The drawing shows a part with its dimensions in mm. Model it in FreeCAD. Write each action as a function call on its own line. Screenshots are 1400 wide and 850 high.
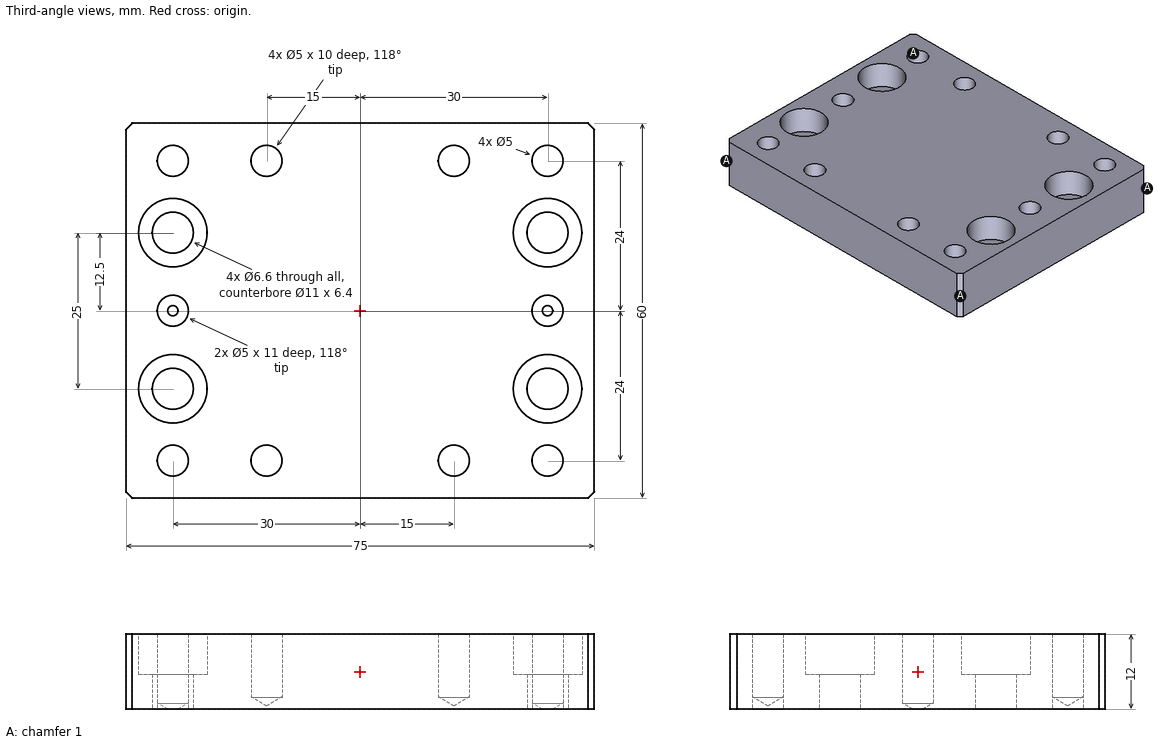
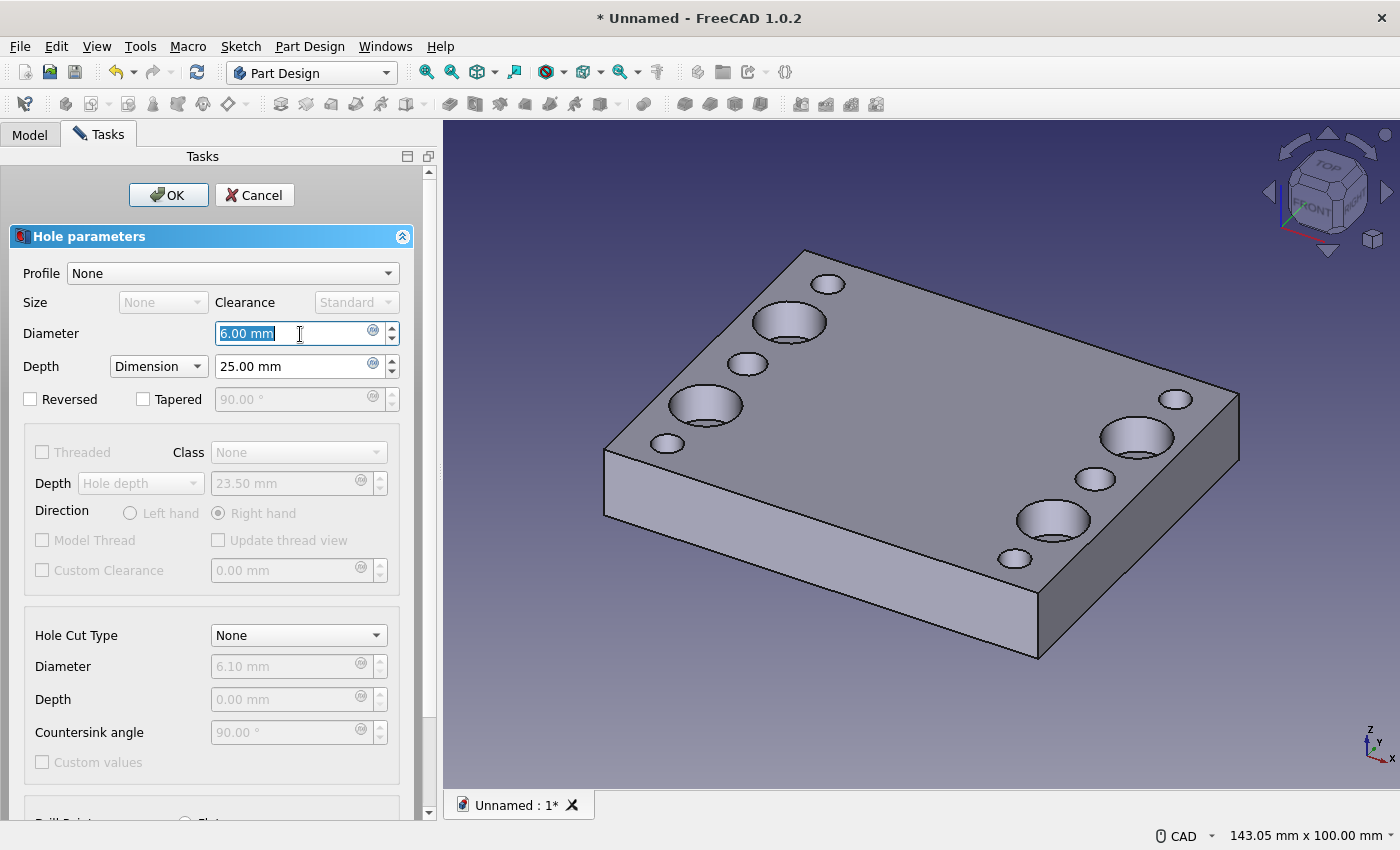
text(5)
key(Tab)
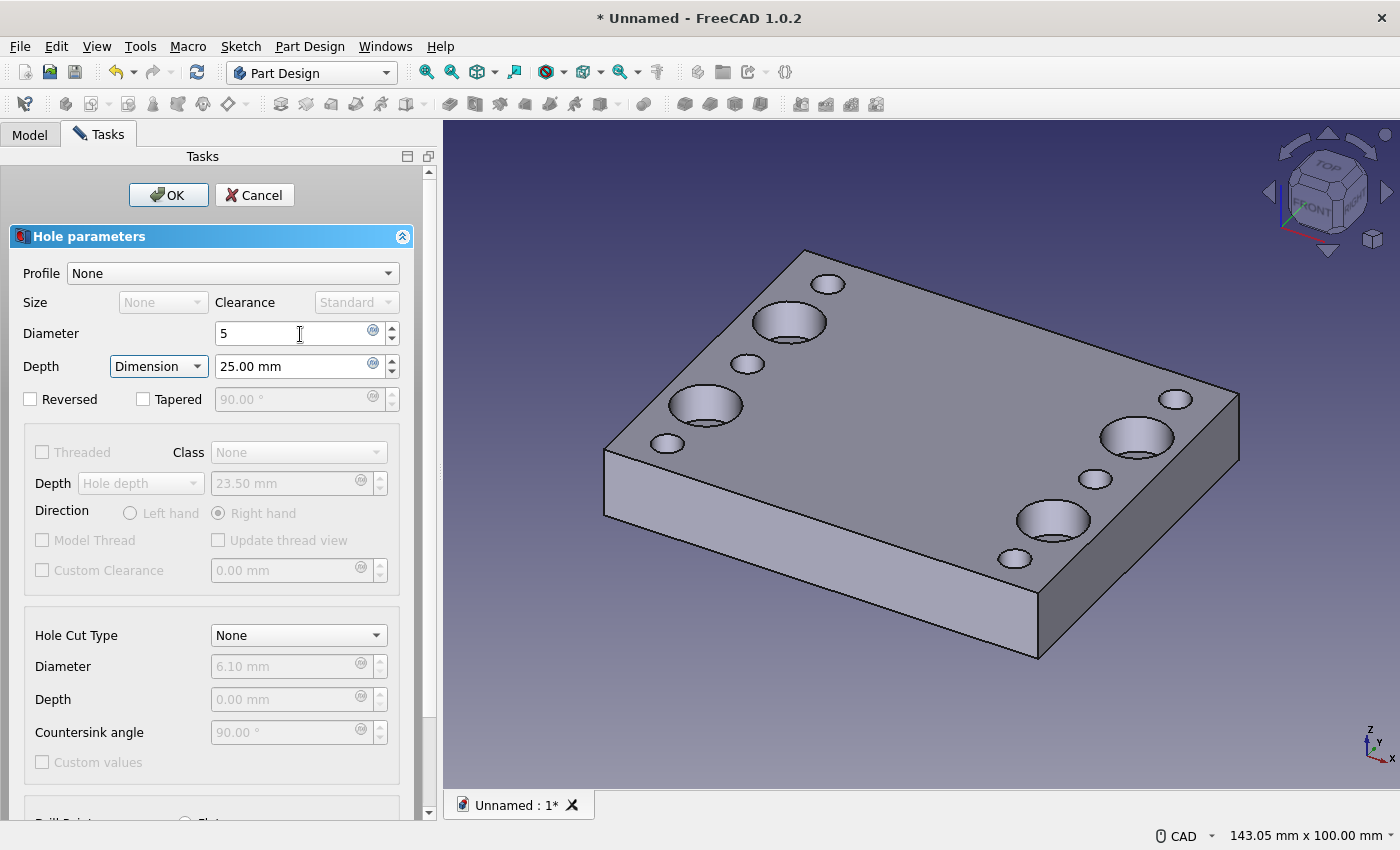
triple_click(300, 366)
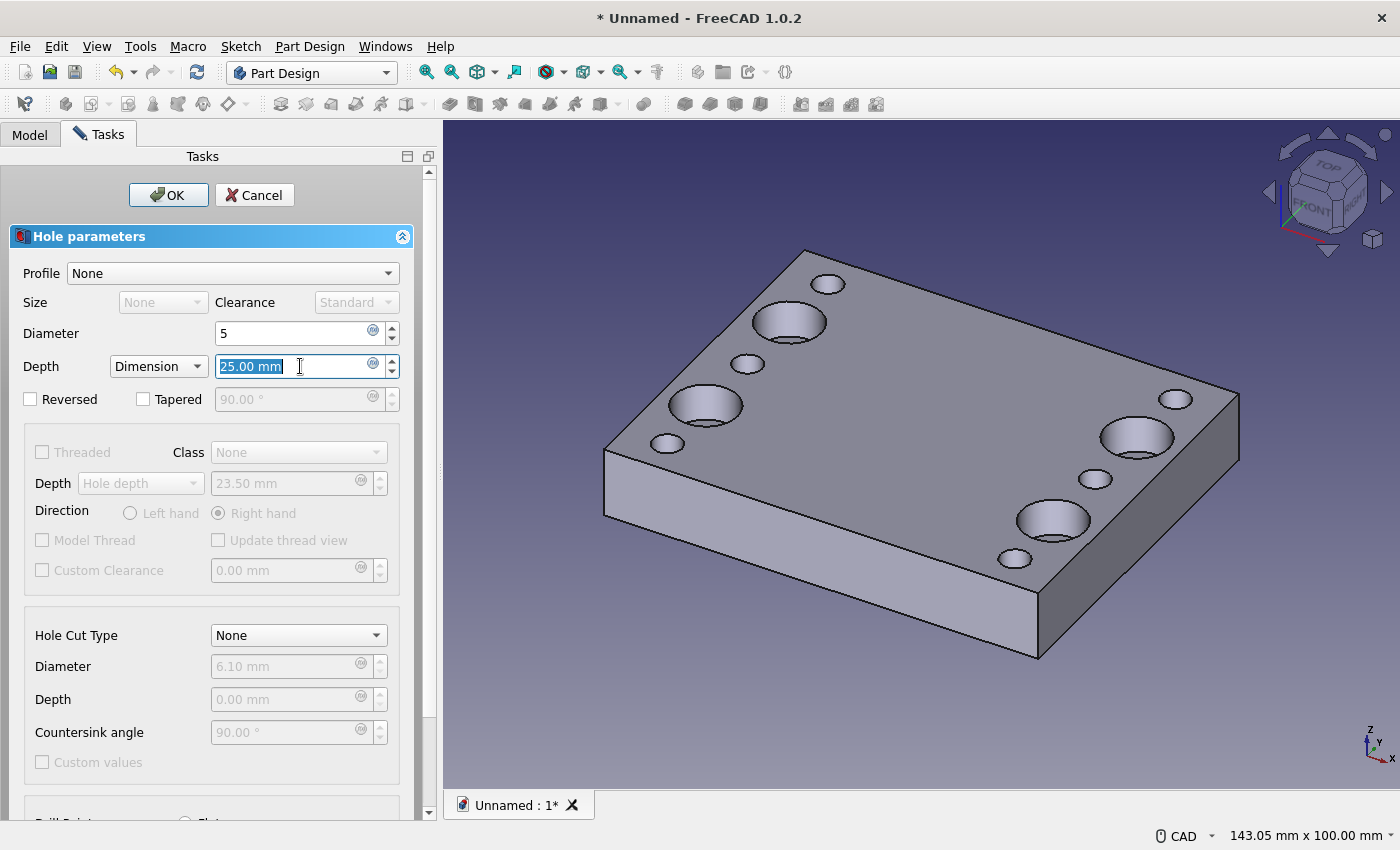
text(11)
key(Tab)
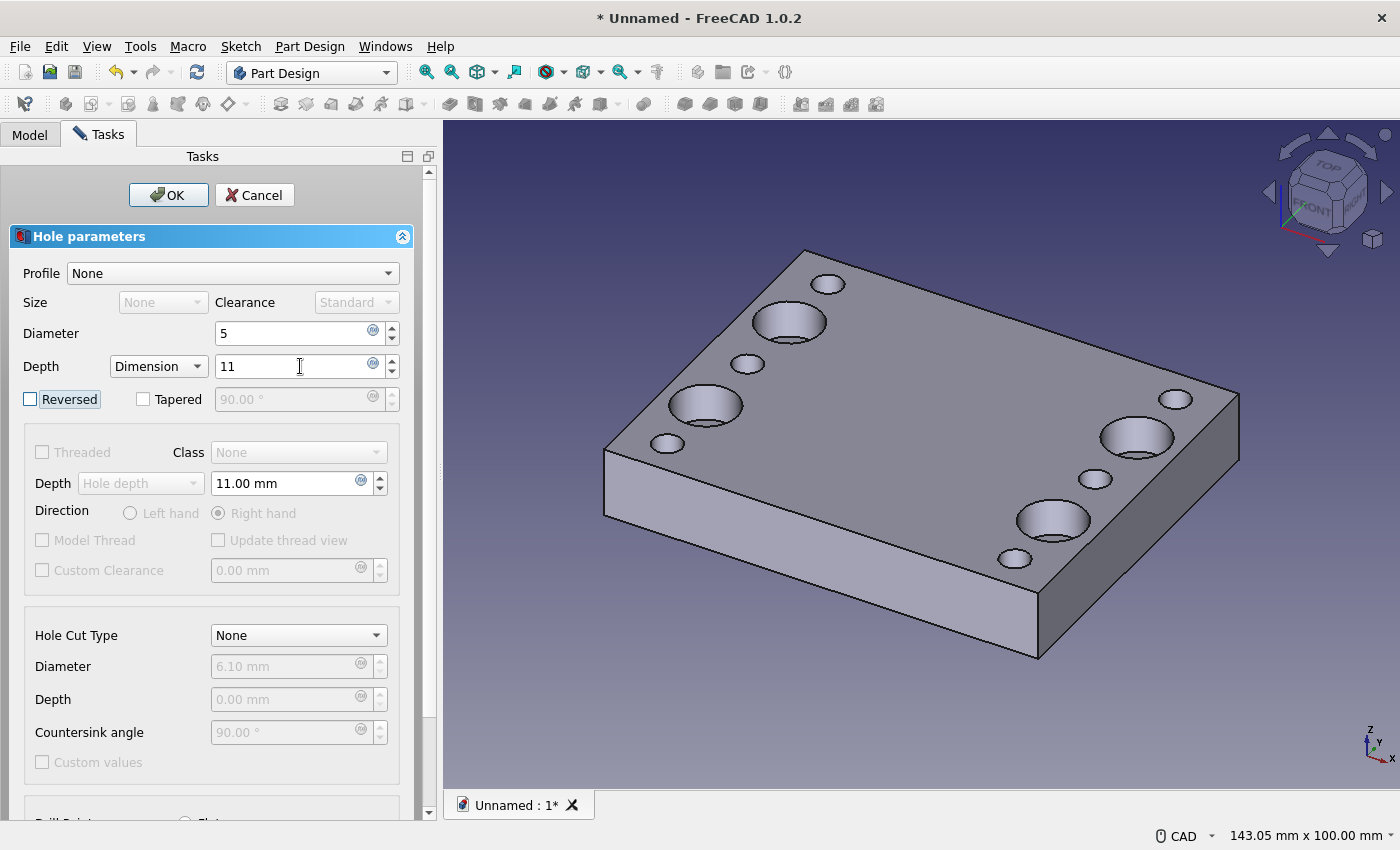
click(169, 195)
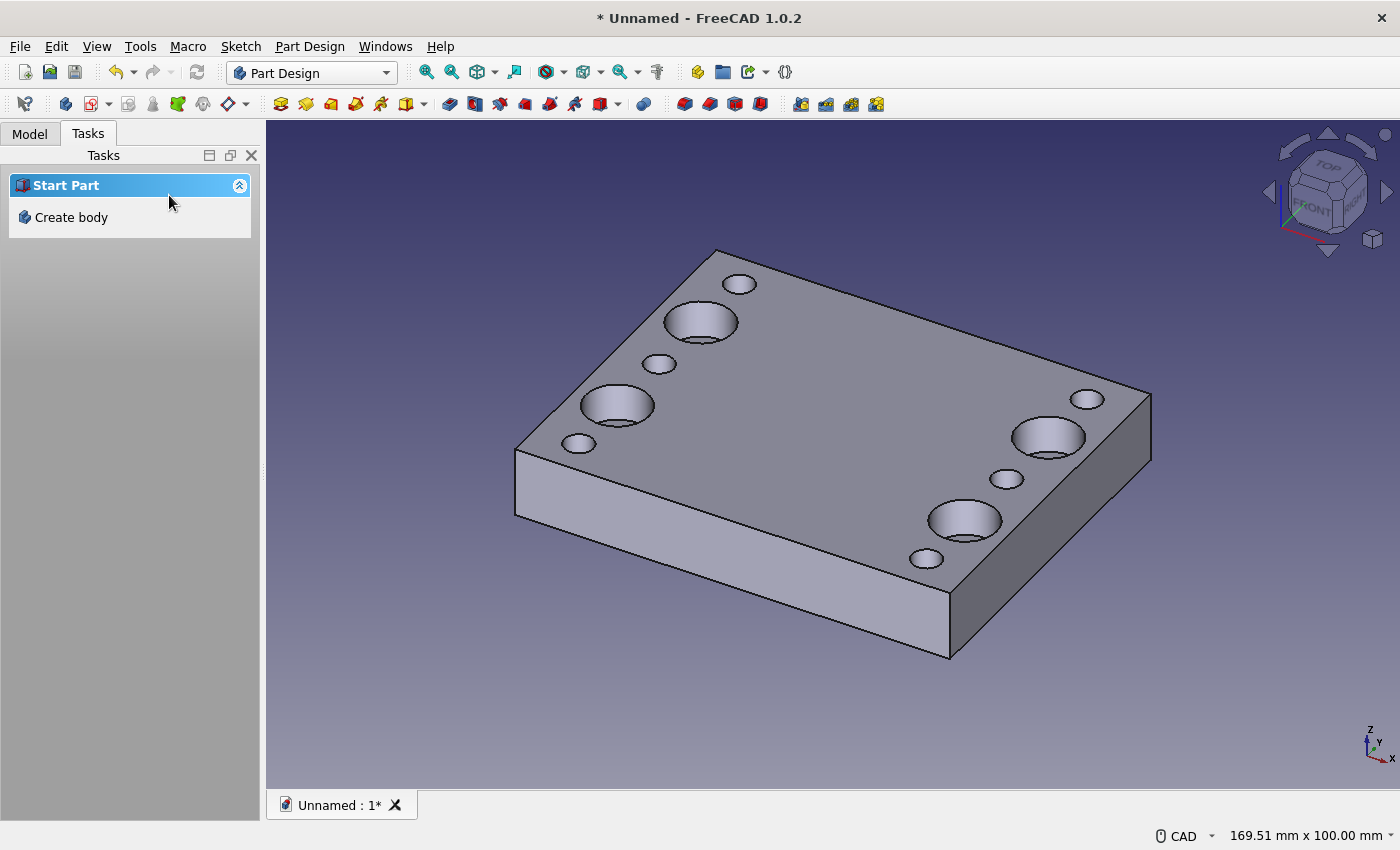
click(833, 421)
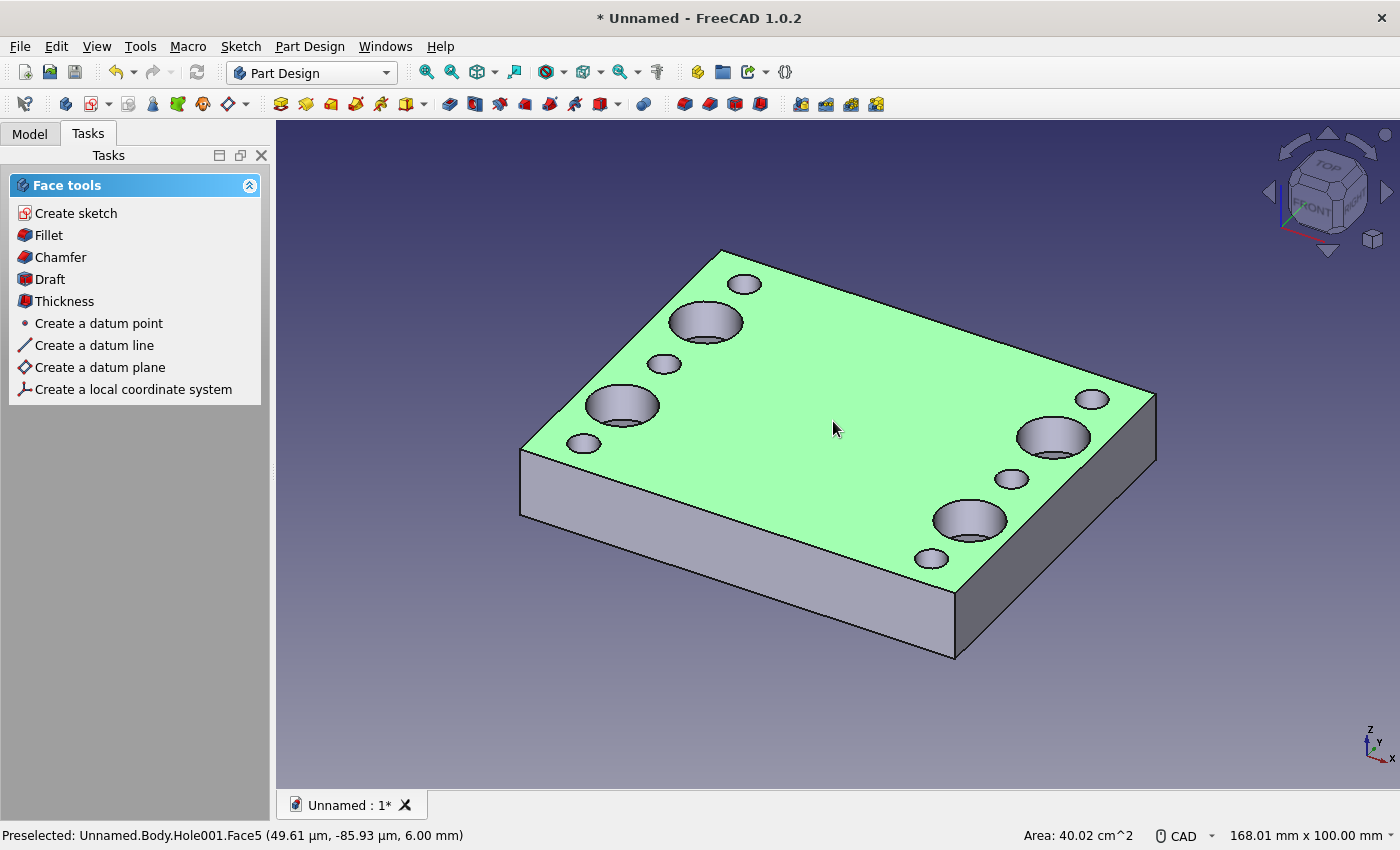
click(90, 104)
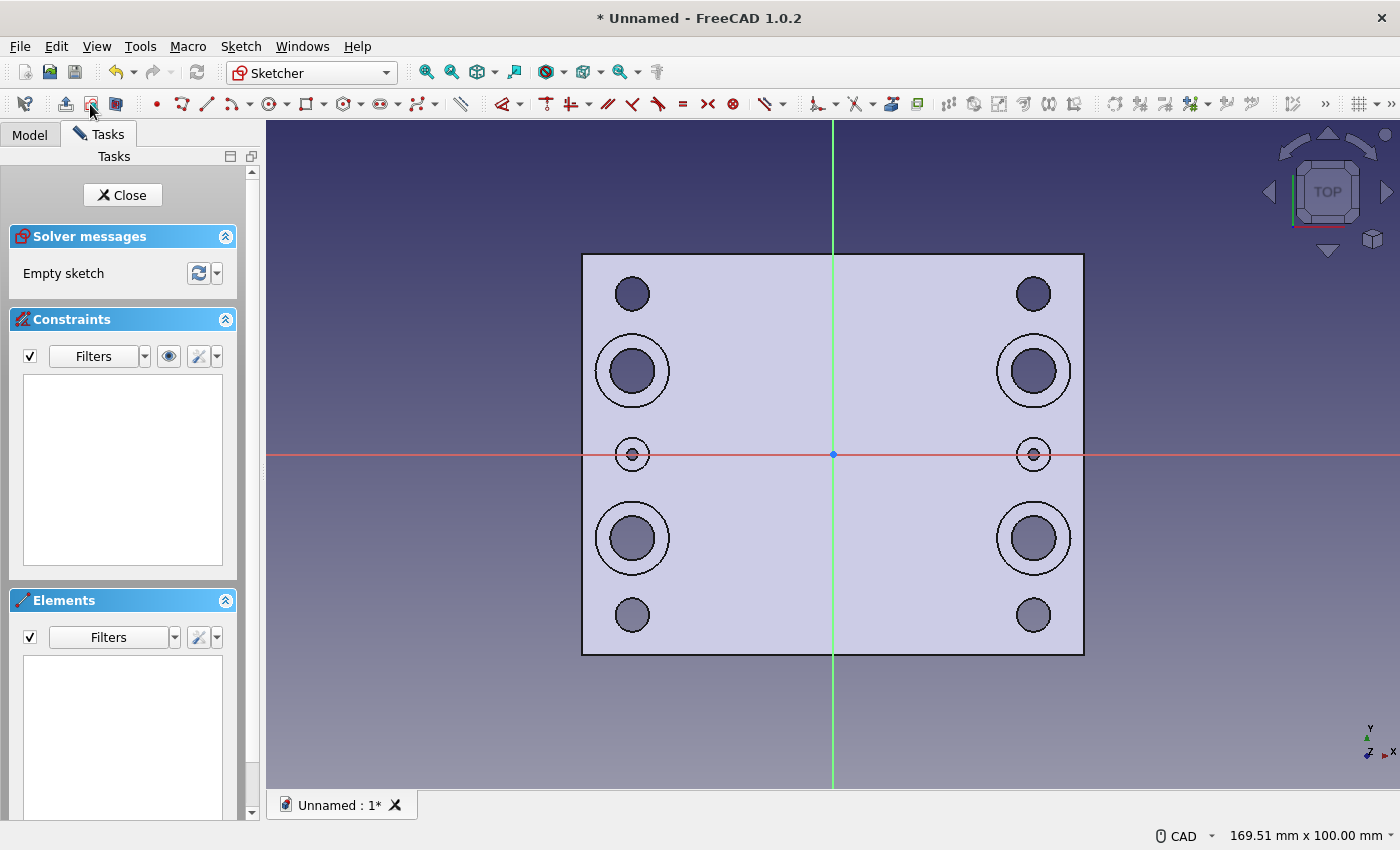
click(268, 104)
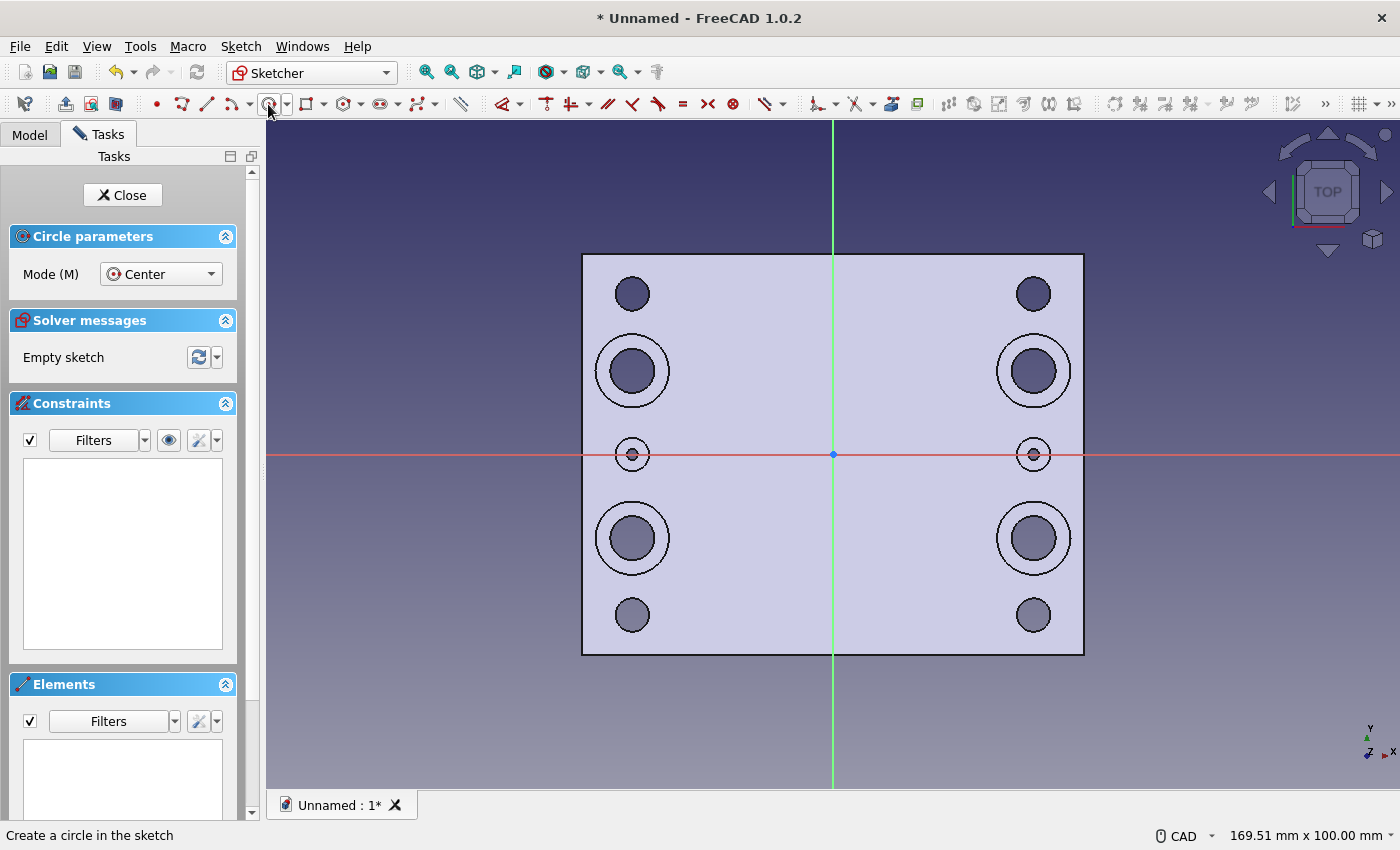
scroll(733, 294, up, 2)